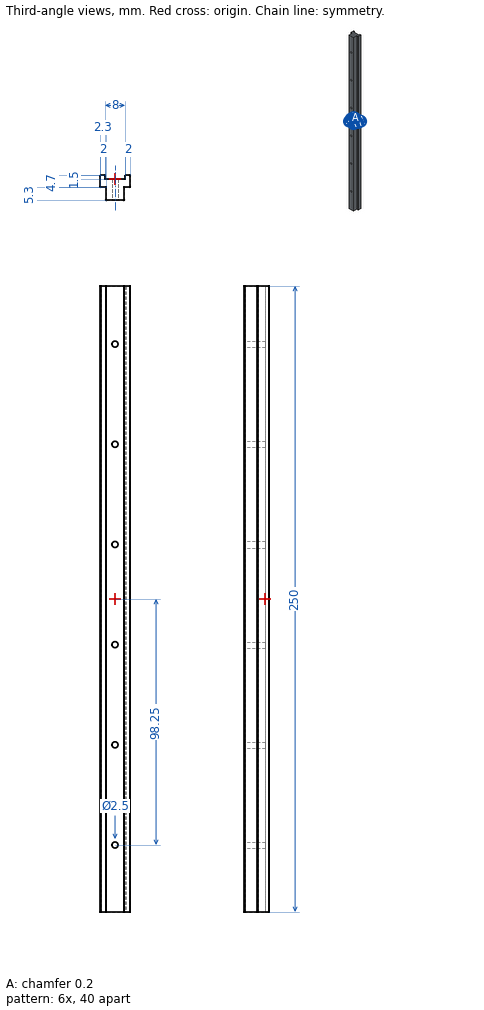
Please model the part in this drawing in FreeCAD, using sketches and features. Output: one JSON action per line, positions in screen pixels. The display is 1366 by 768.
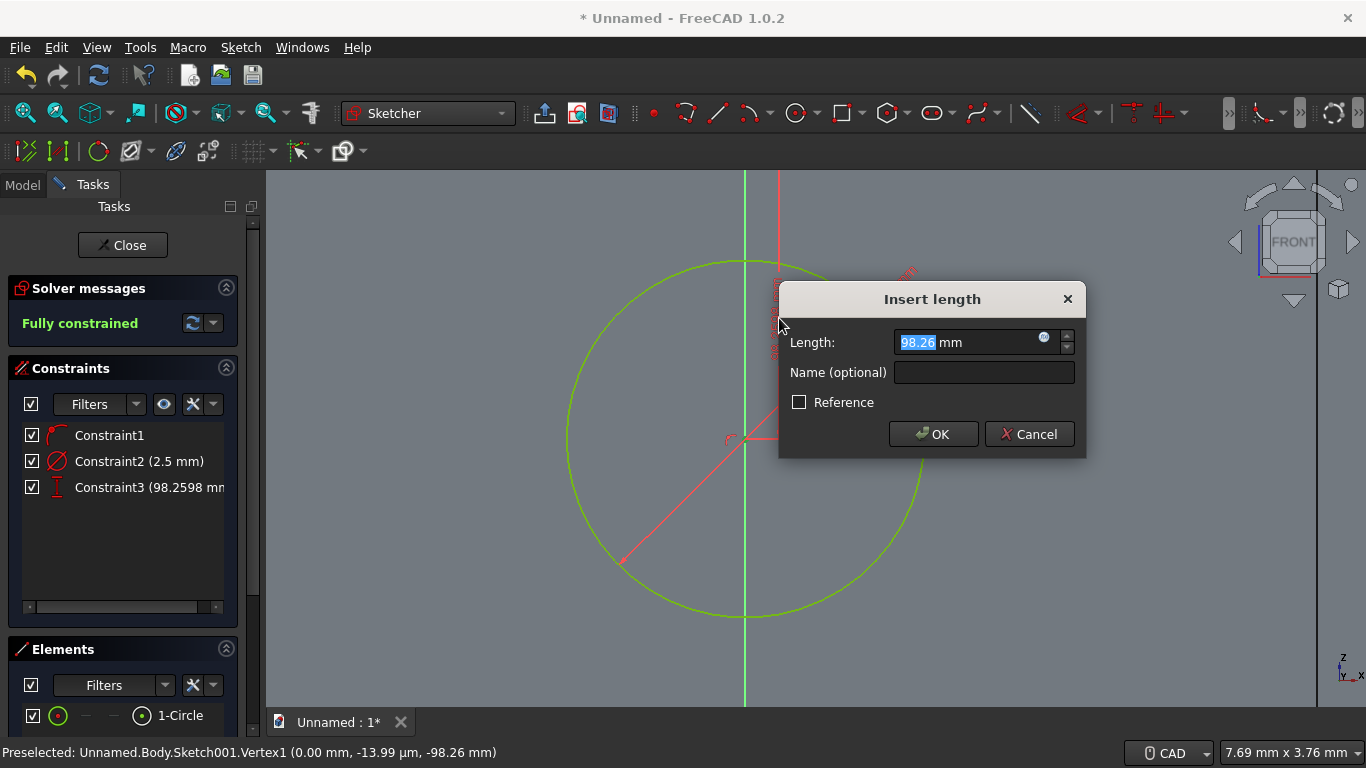
{"action": "type", "text": "98.25"}
{"action": "key", "text": "Return"}
{"action": "key", "text": "Escape"}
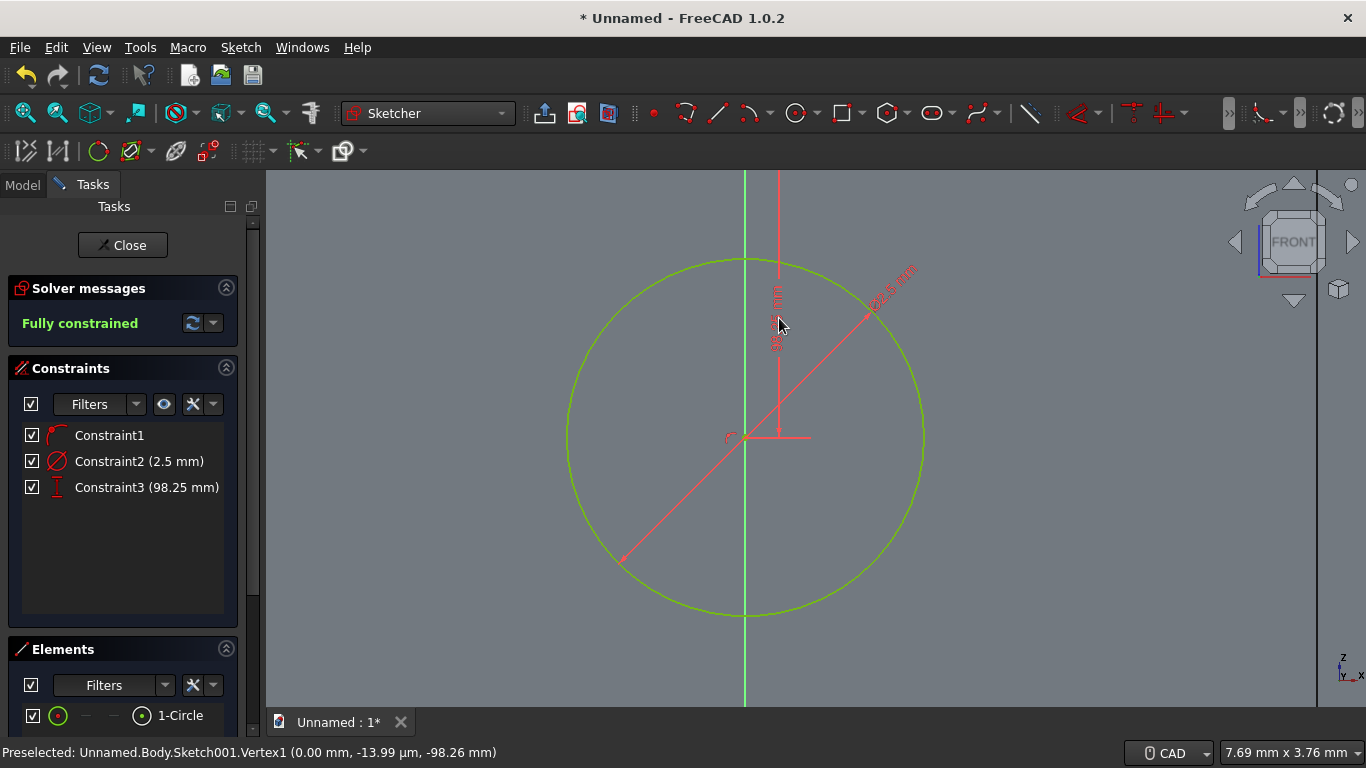
{"action": "left_click", "coordinate": [123, 245]}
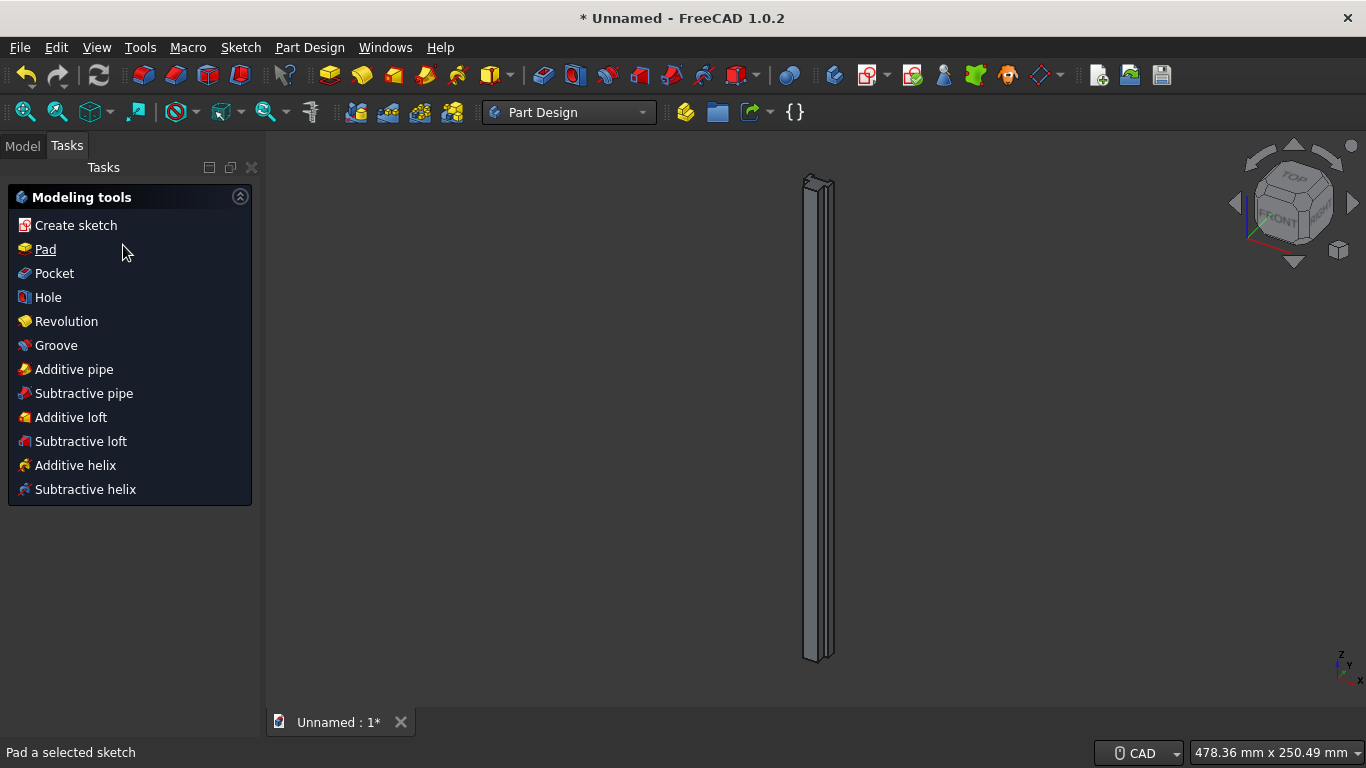
{"action": "left_click", "coordinate": [544, 76]}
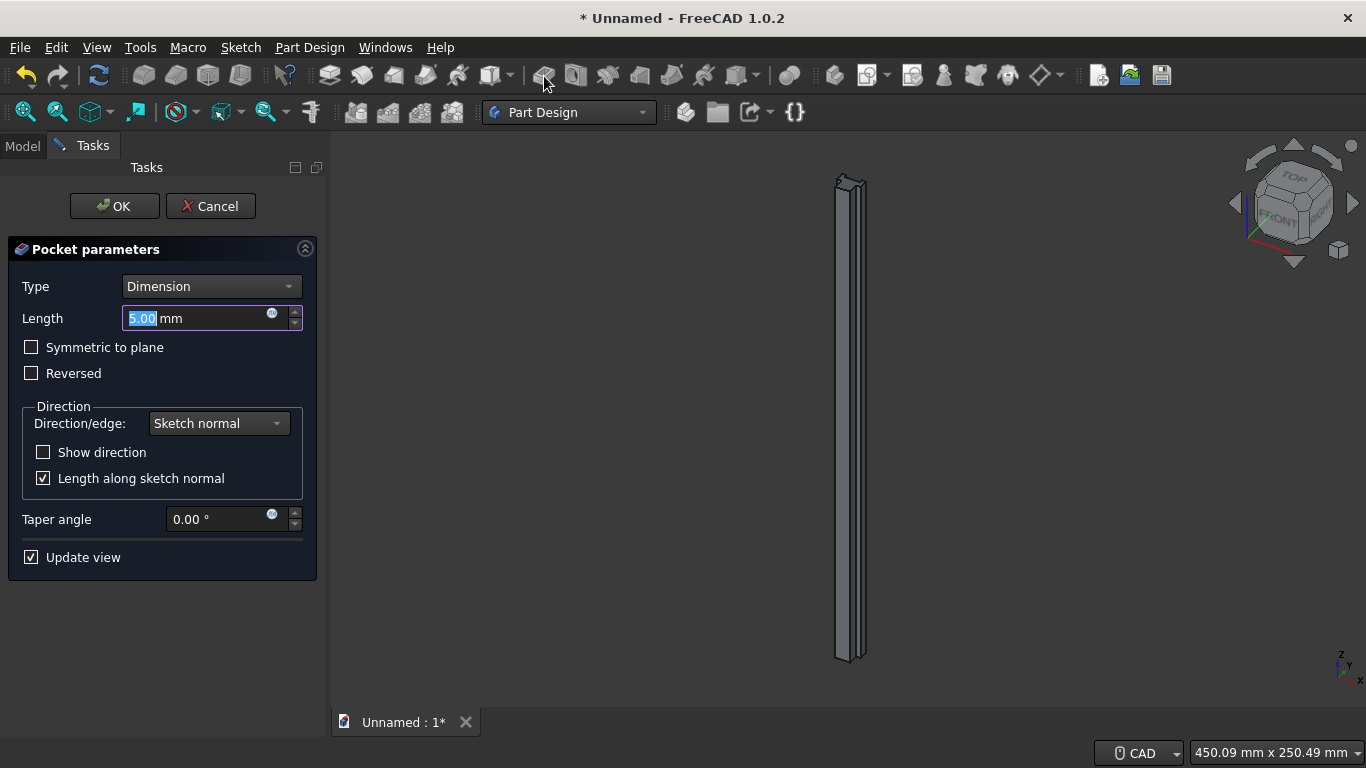
{"action": "left_click", "coordinate": [212, 286]}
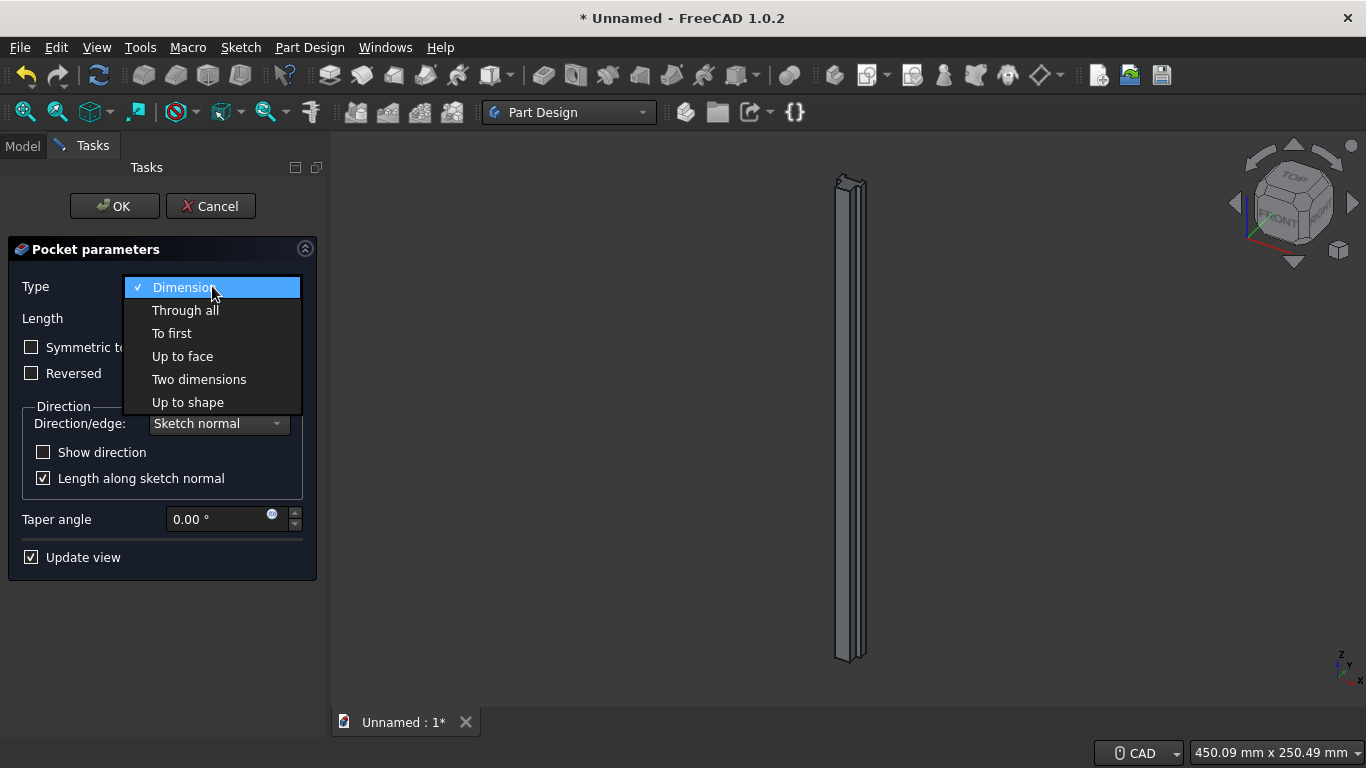
{"action": "left_click", "coordinate": [212, 310]}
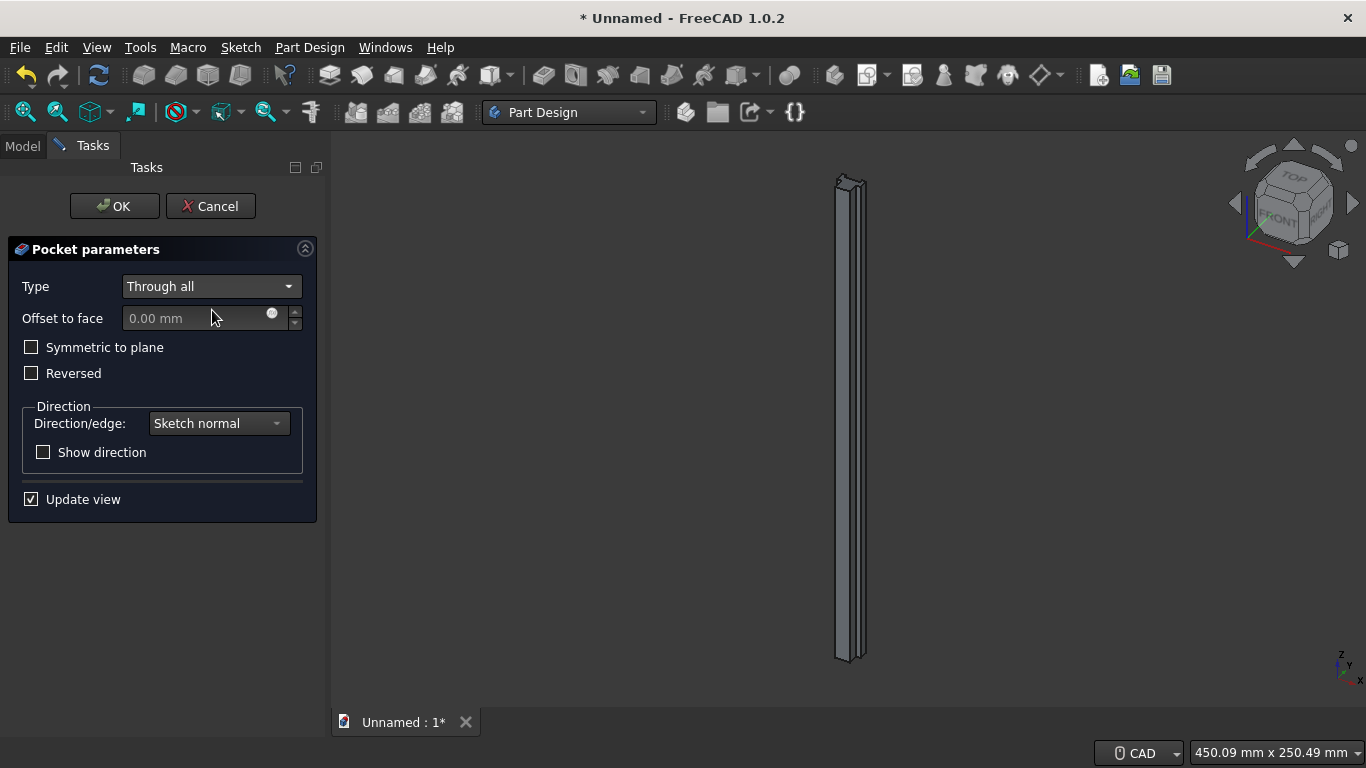
{"action": "left_click", "coordinate": [30, 373]}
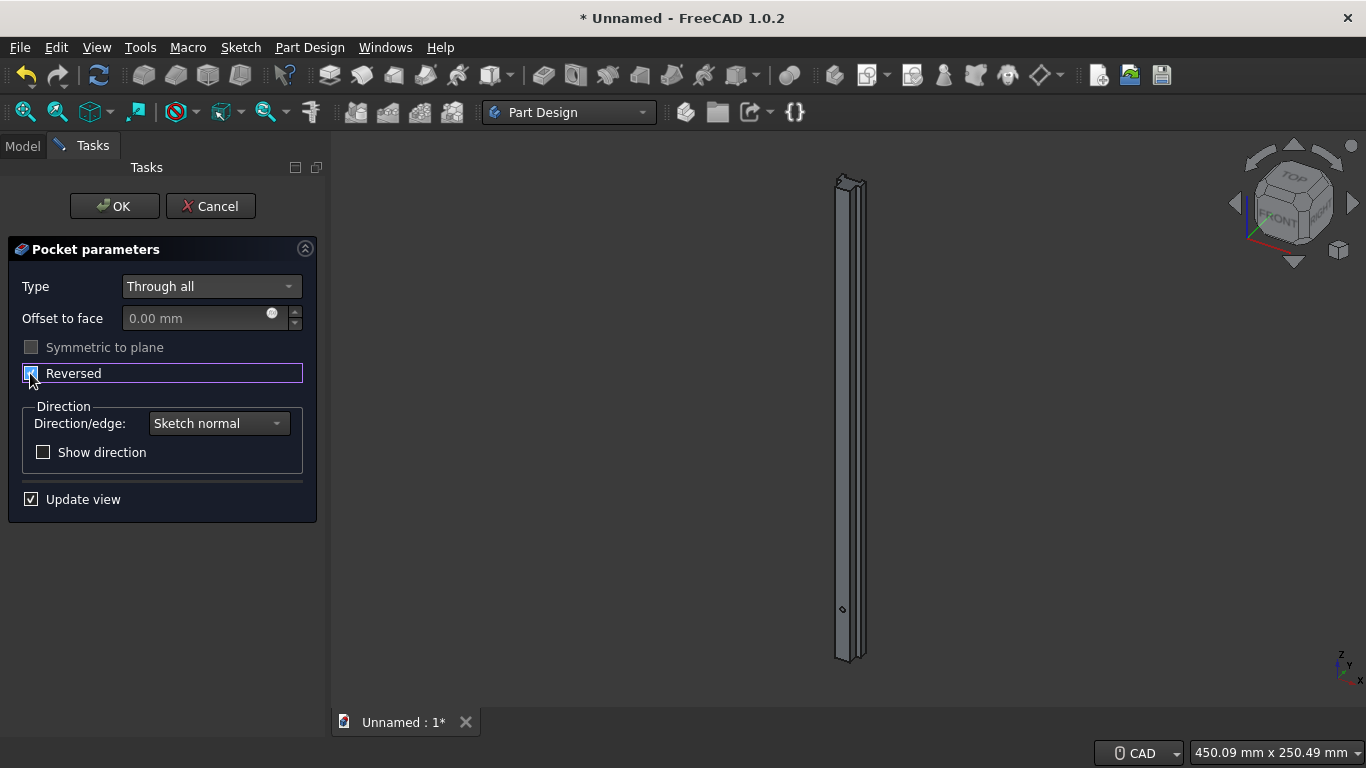
{"action": "left_click", "coordinate": [115, 206]}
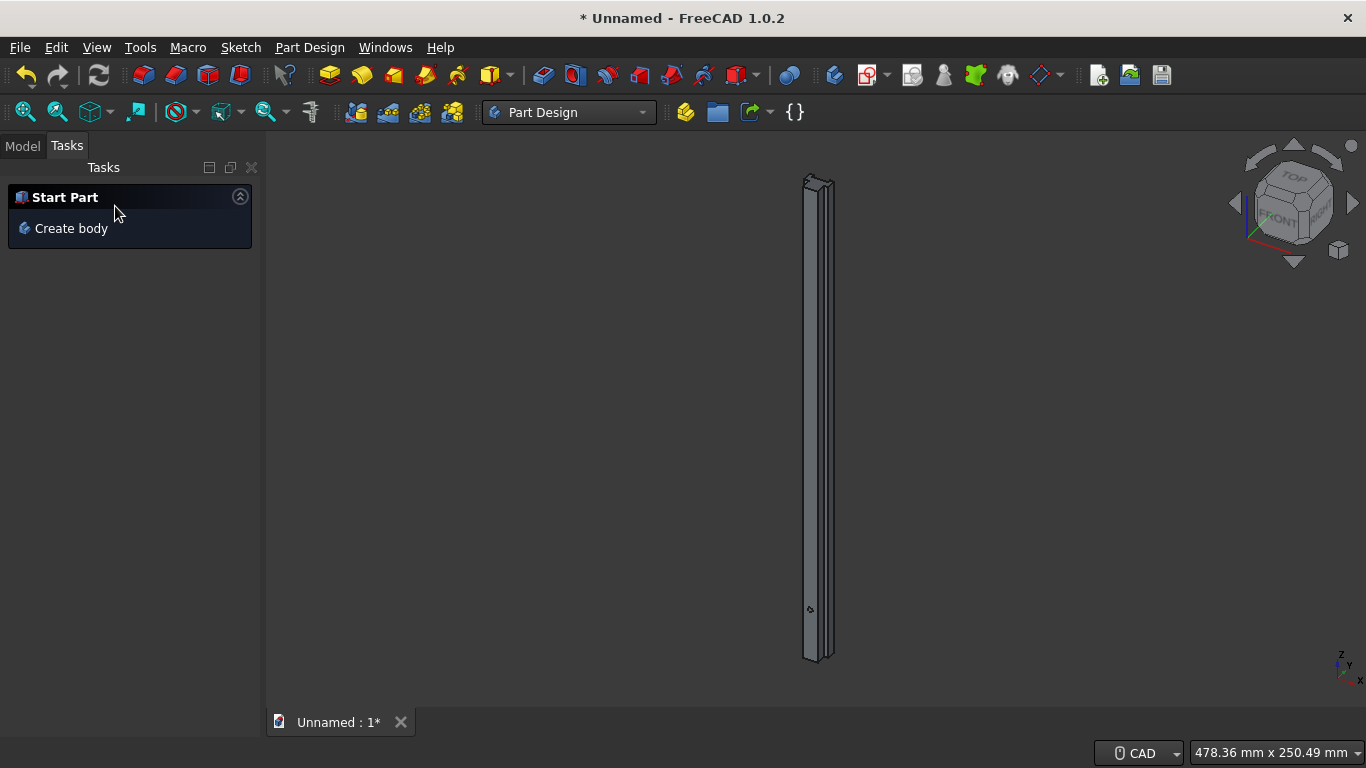
{"action": "left_click", "coordinate": [828, 422]}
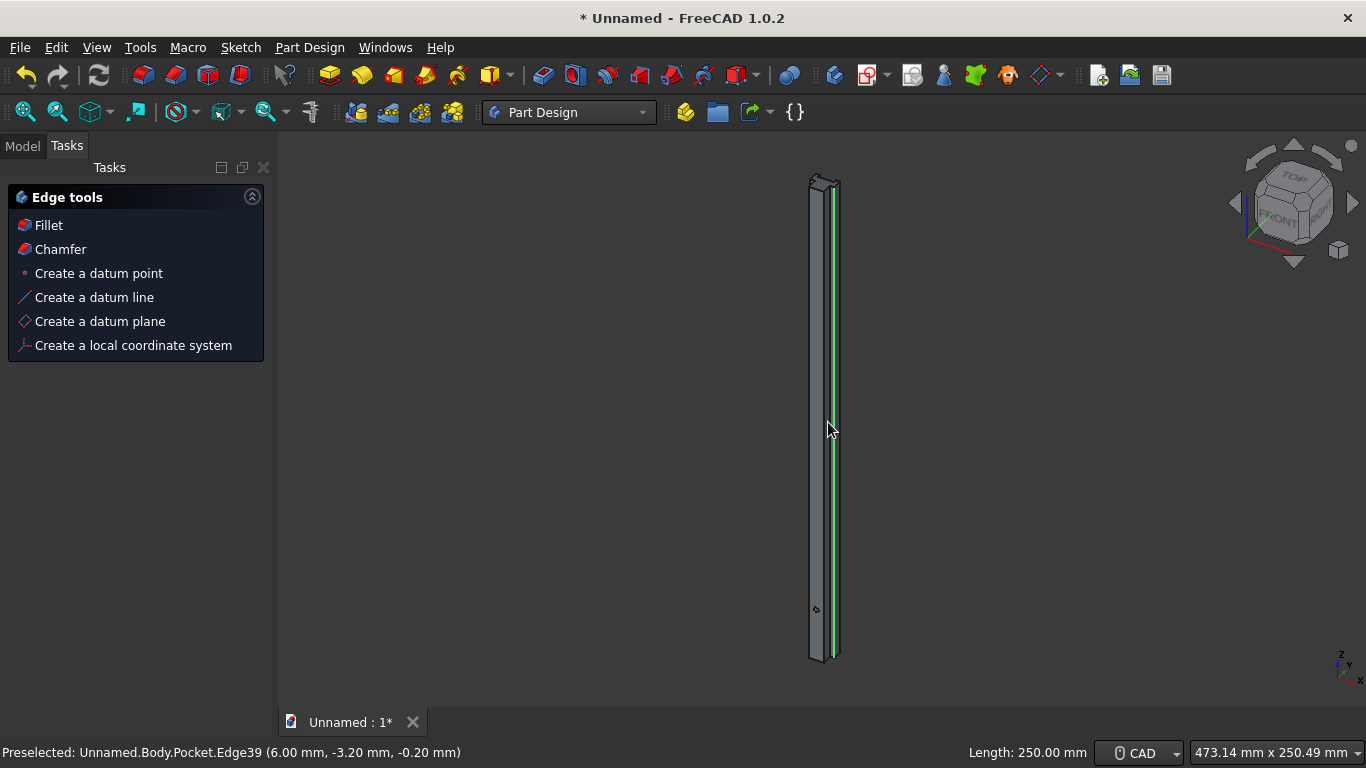
{"action": "left_click", "coordinate": [824, 426], "text": "ctrl"}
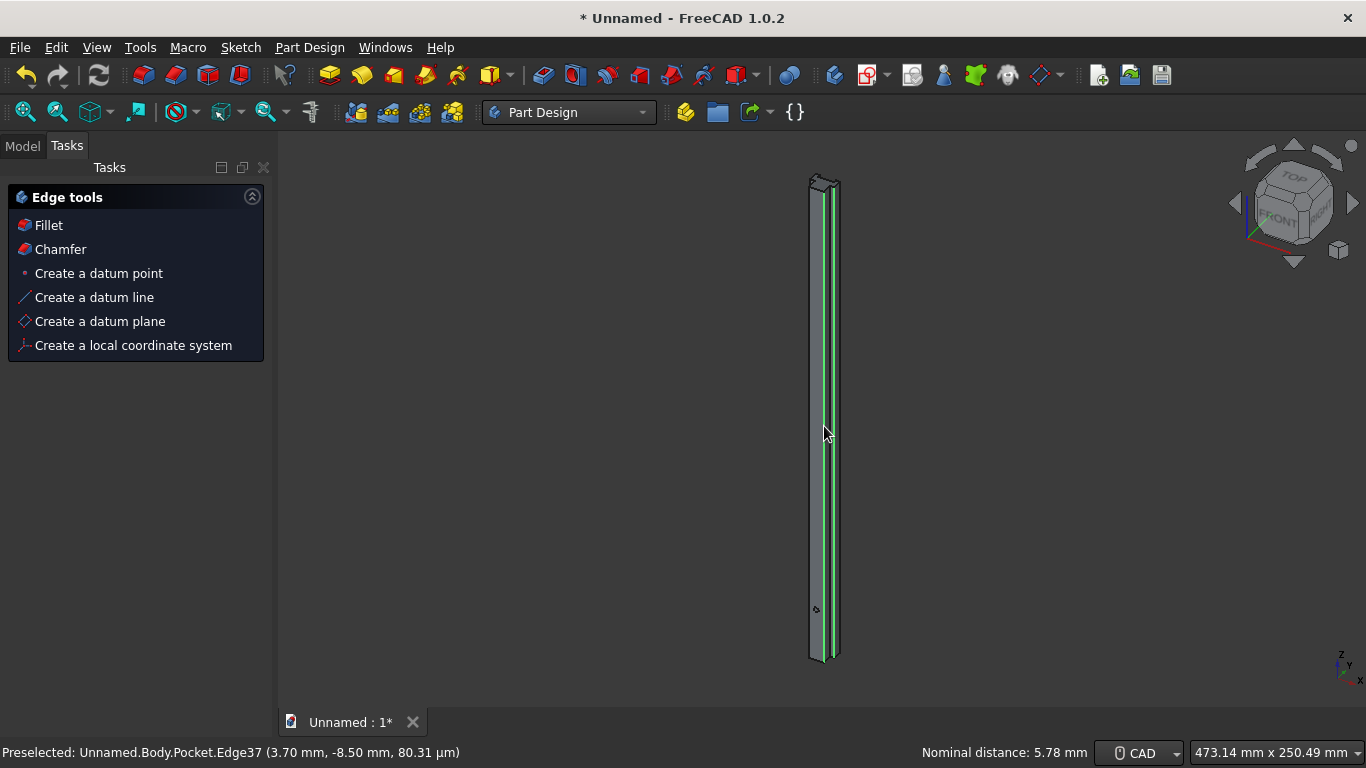
{"action": "key", "text": "0"}